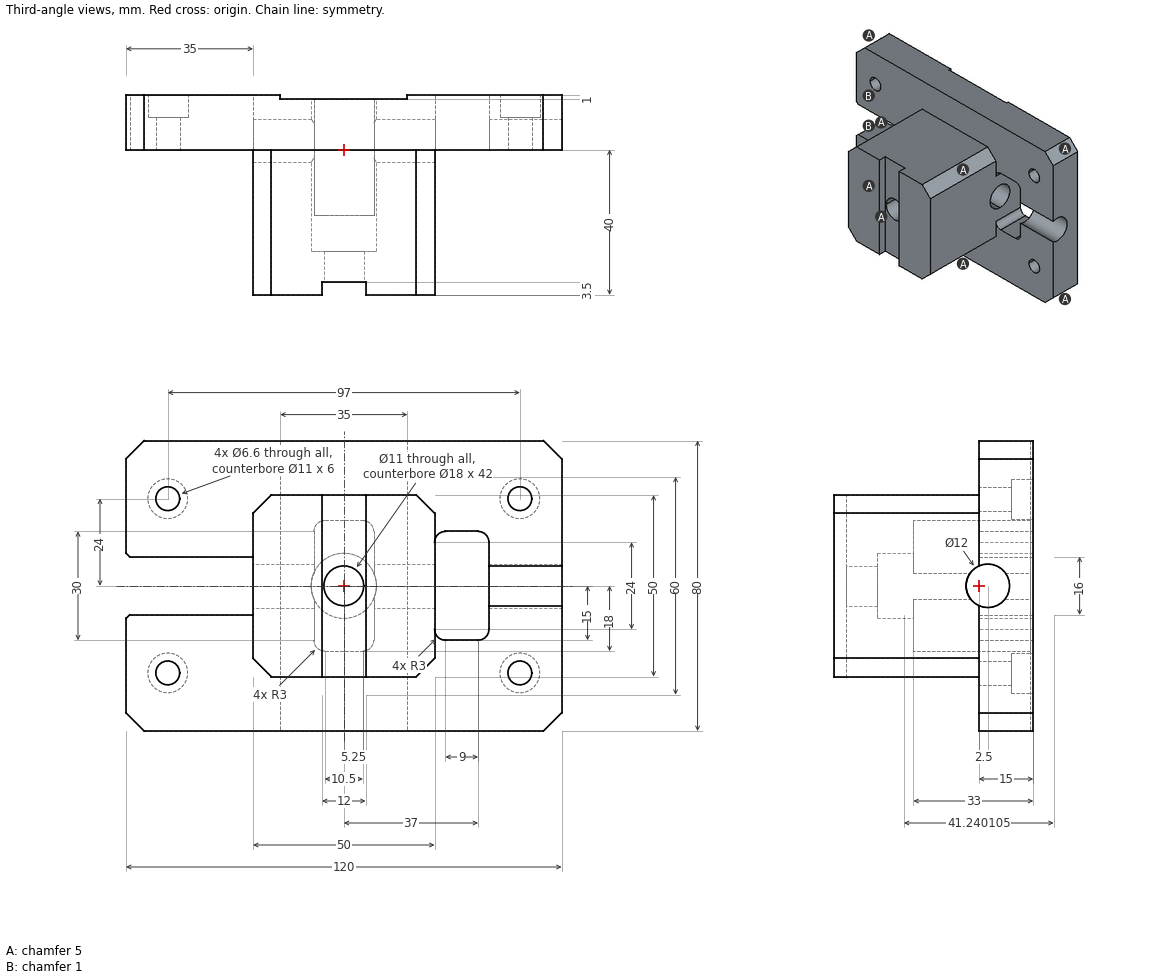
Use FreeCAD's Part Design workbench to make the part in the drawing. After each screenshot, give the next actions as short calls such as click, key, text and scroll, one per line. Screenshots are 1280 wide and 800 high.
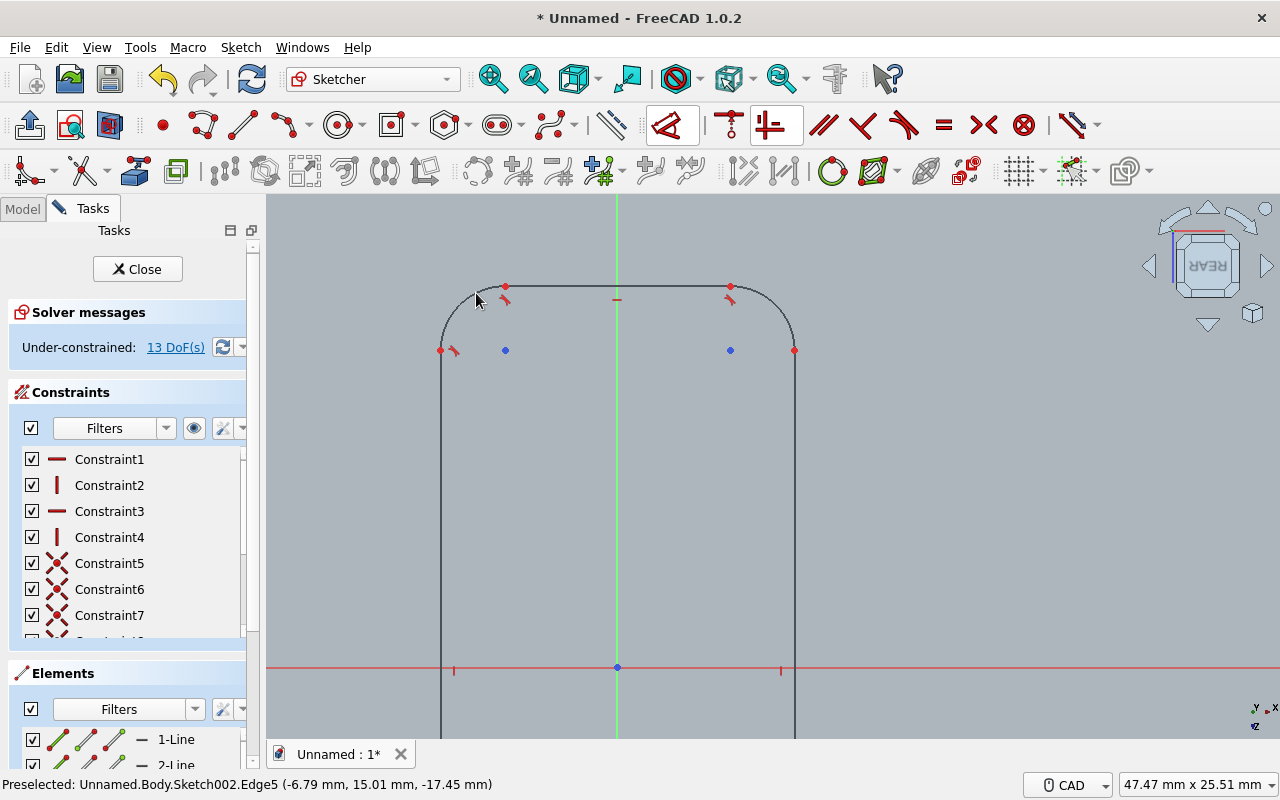
click(441, 542)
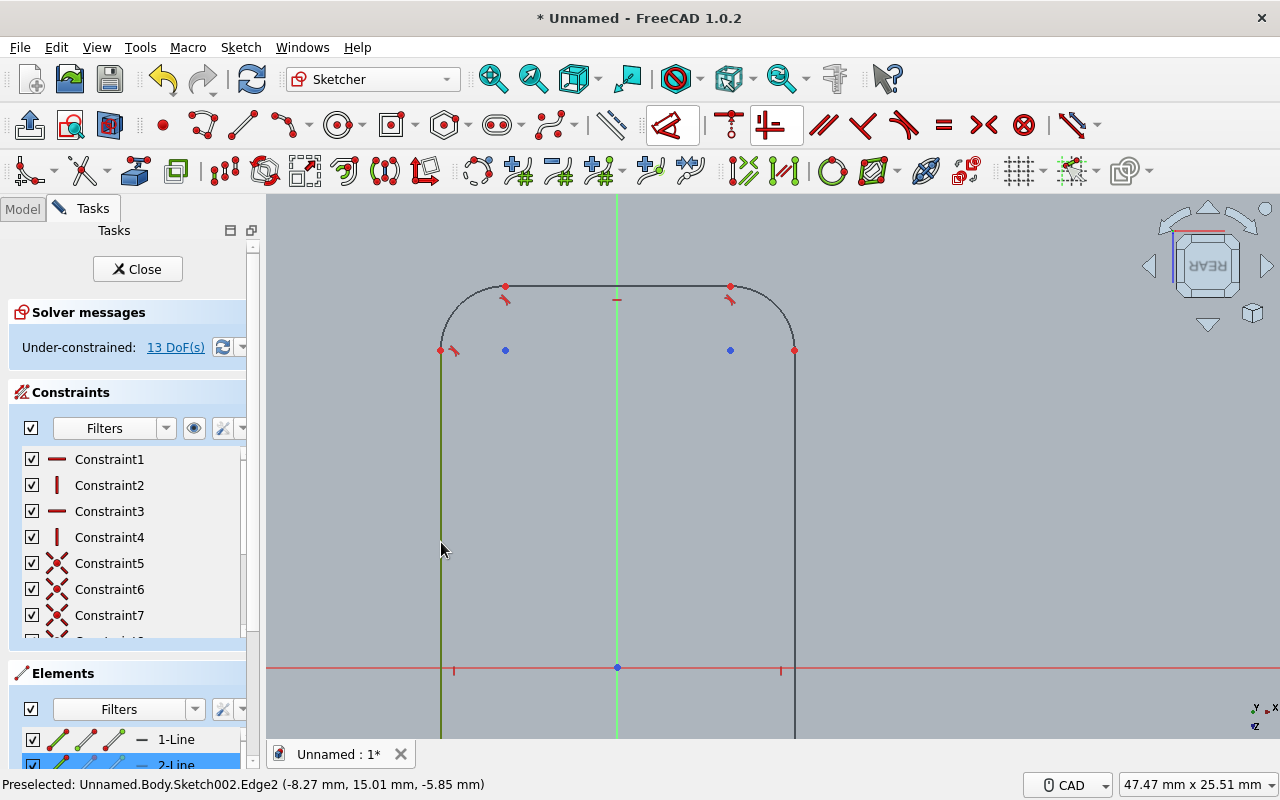
scroll(776, 302, down, 4)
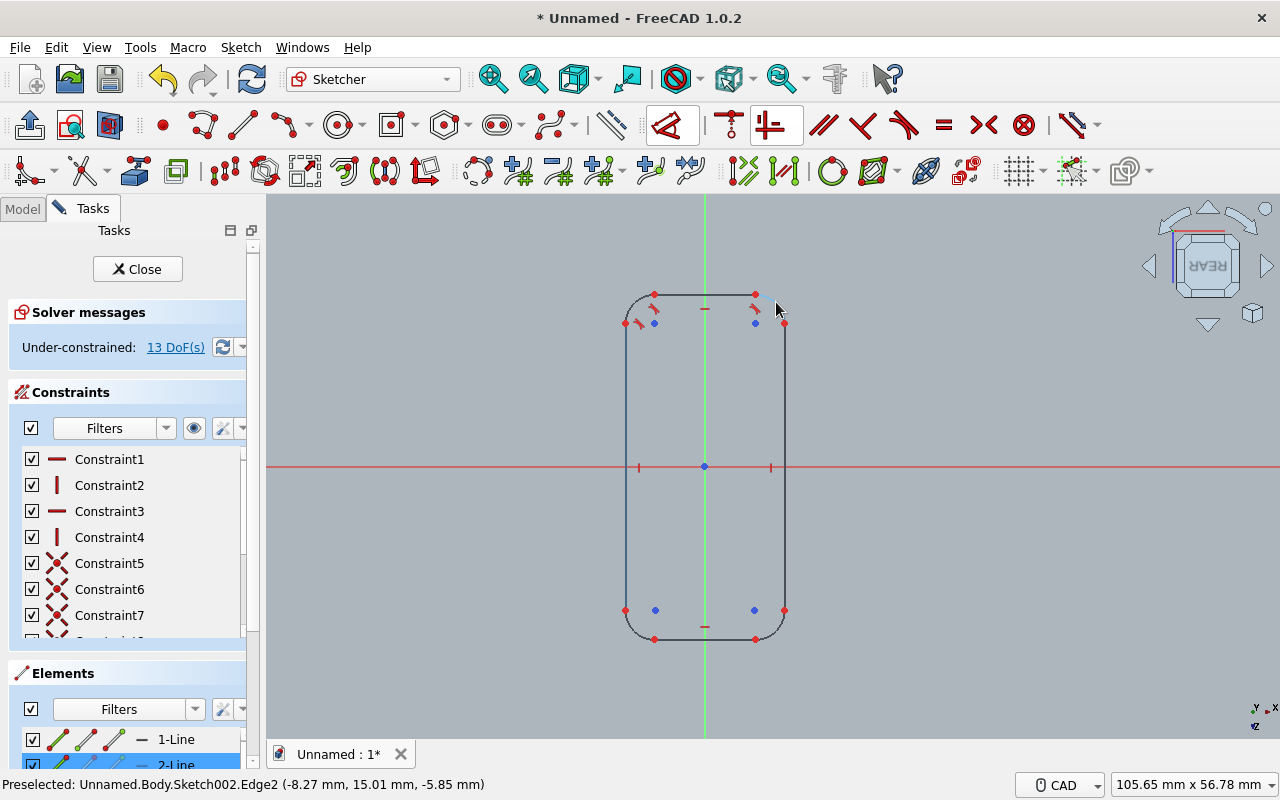
click(629, 624)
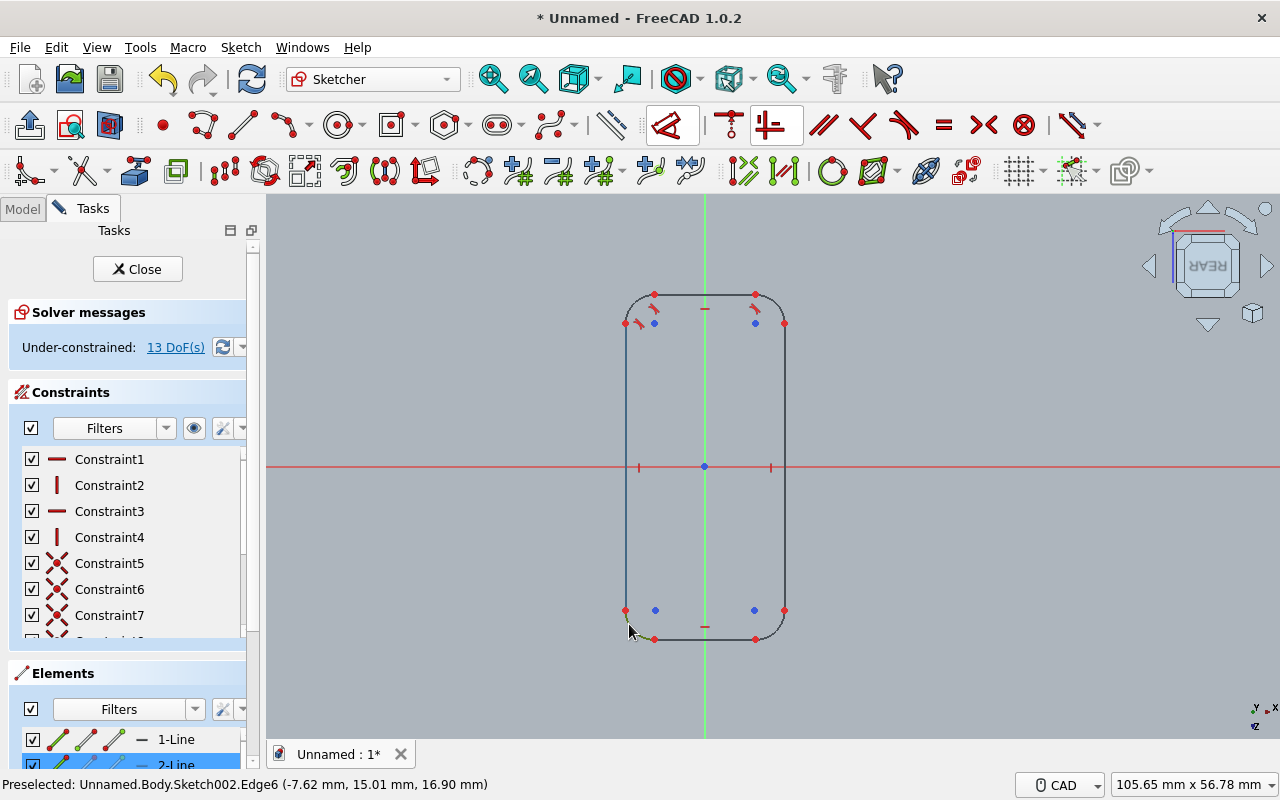
click(904, 126)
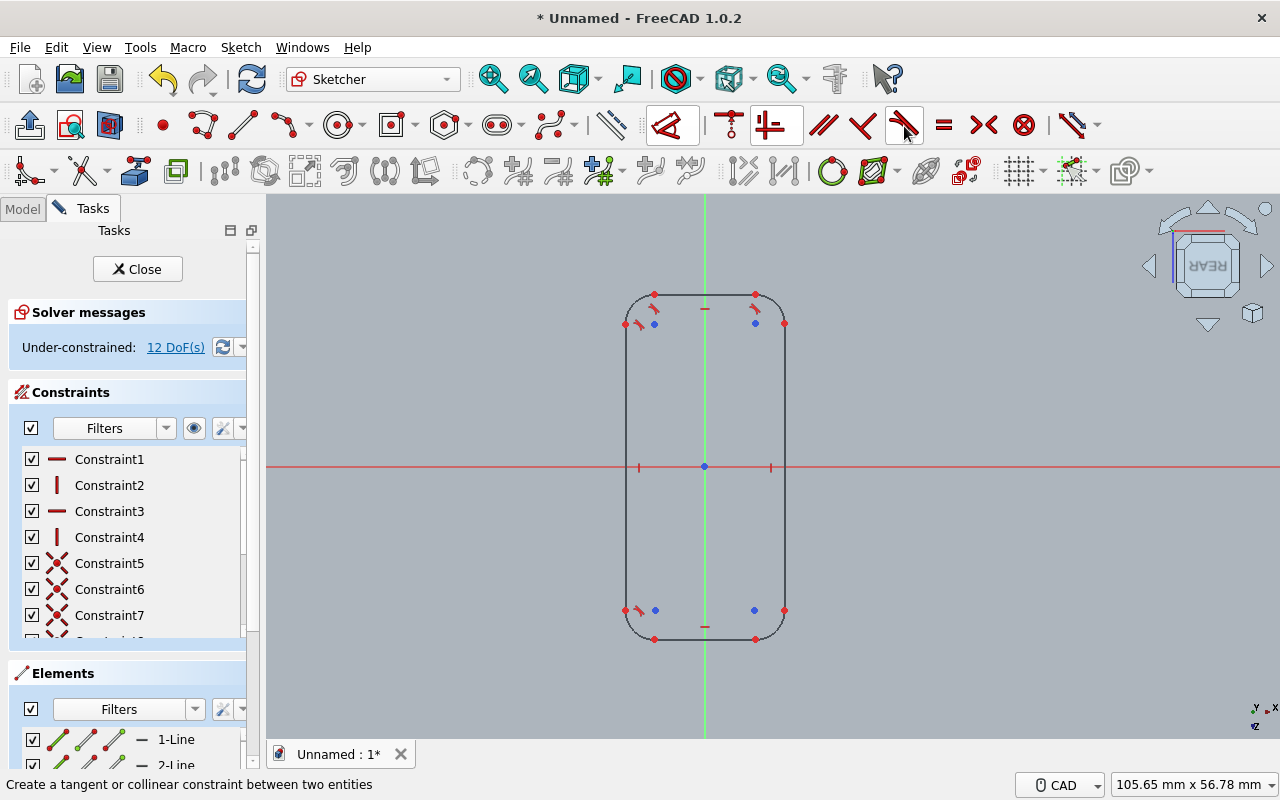
click(685, 640)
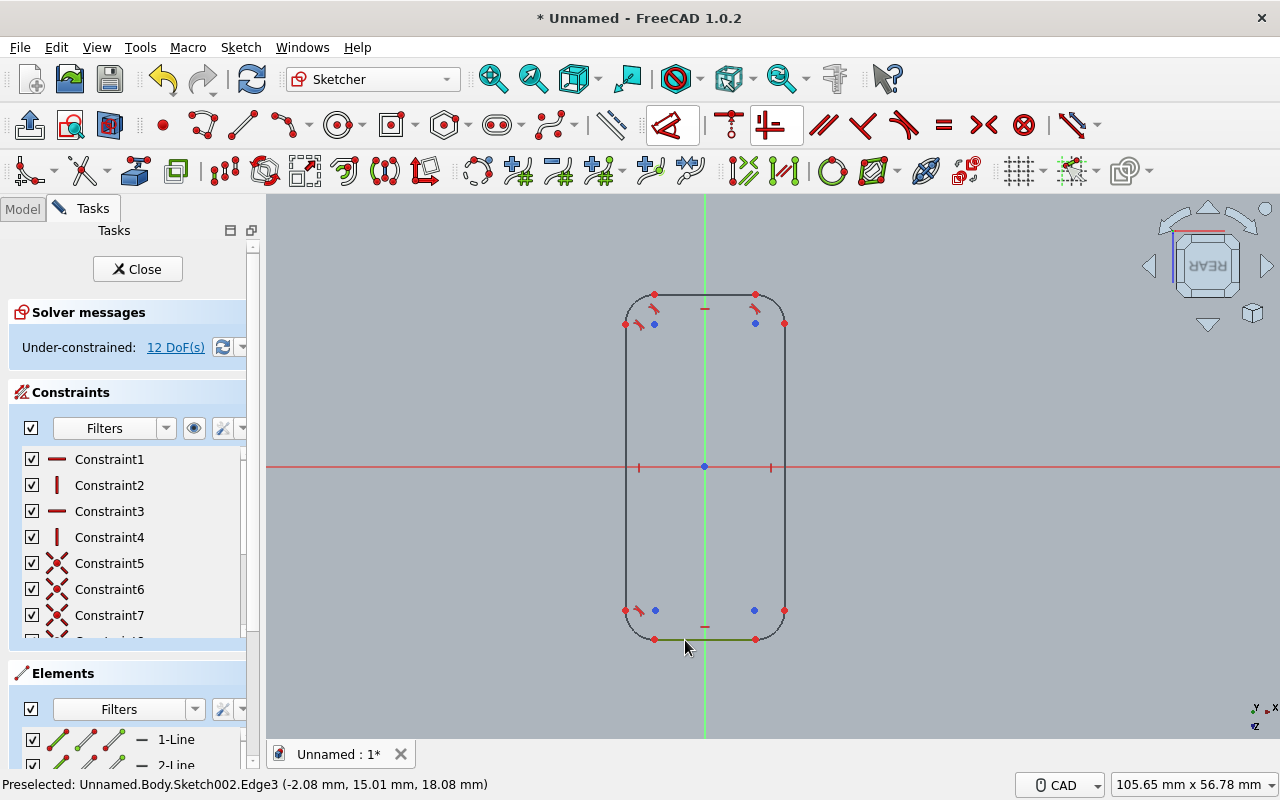
click(629, 624)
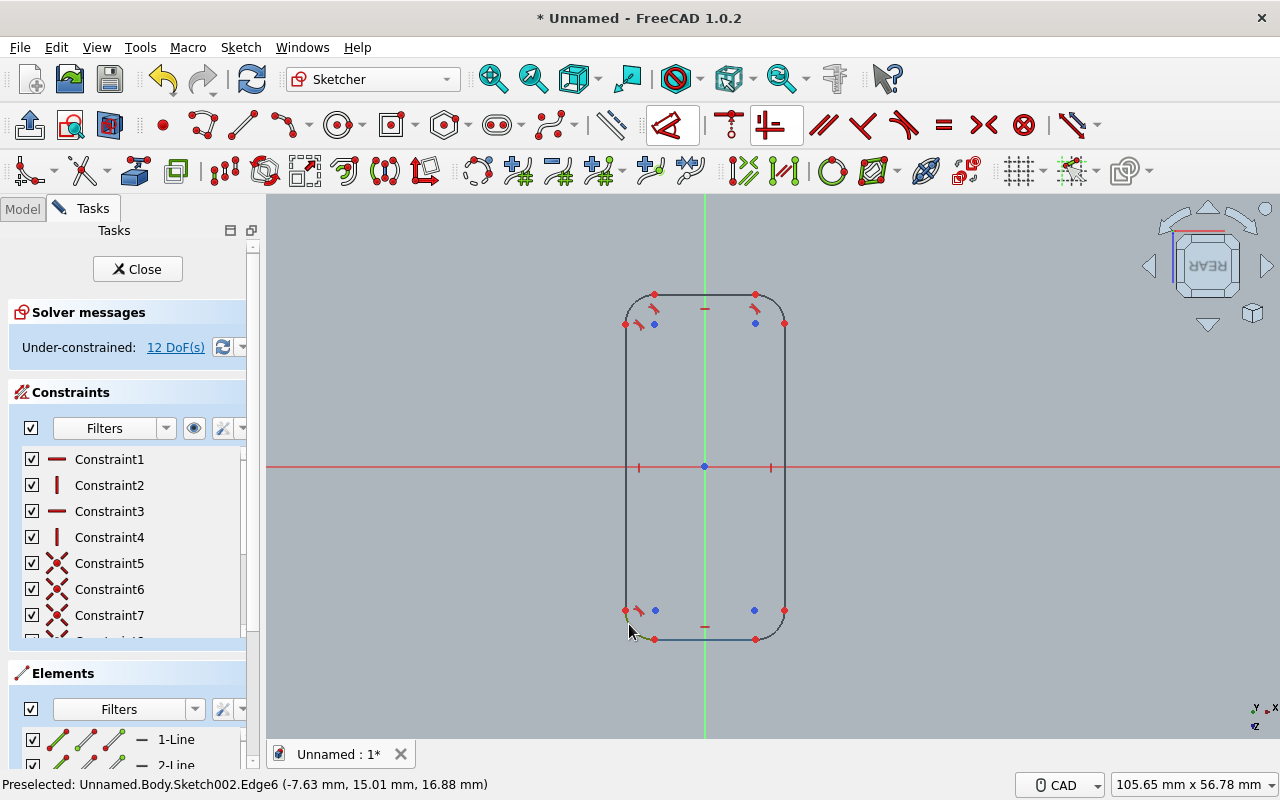
click(904, 126)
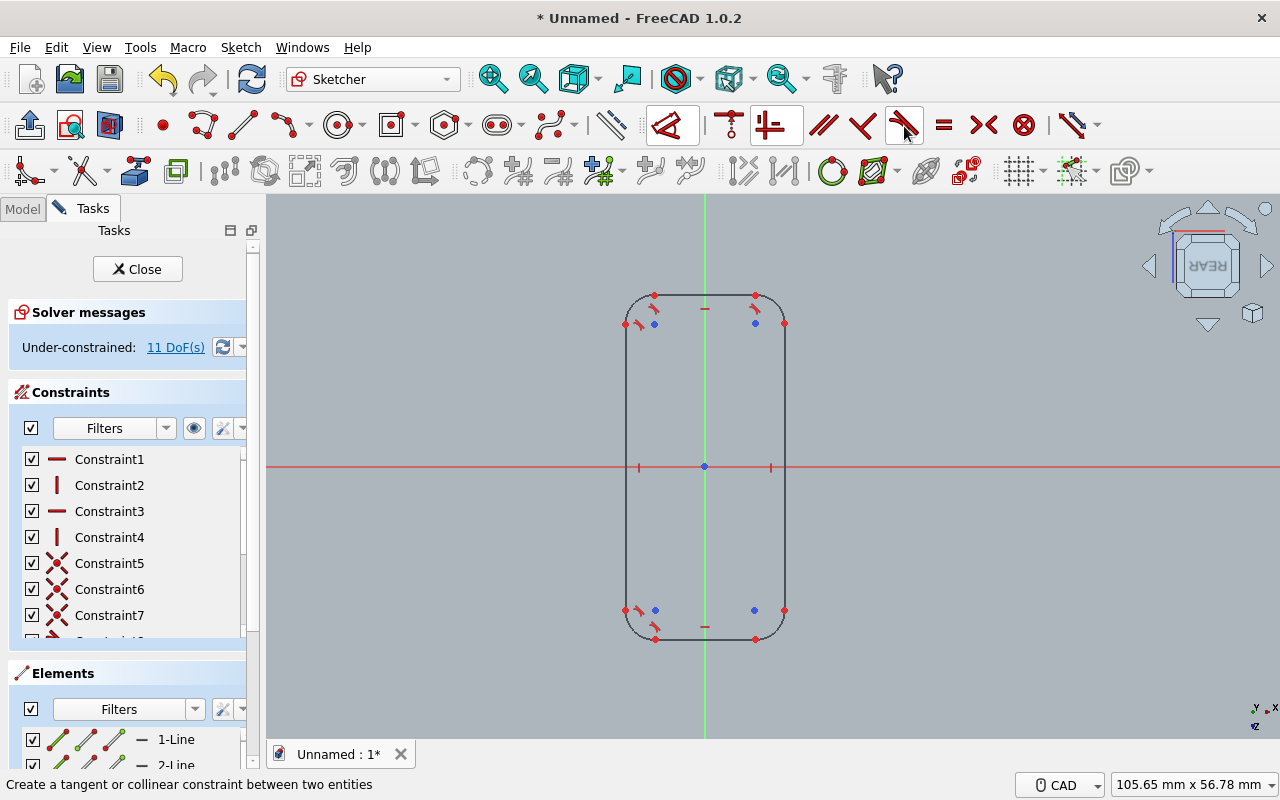
click(685, 640)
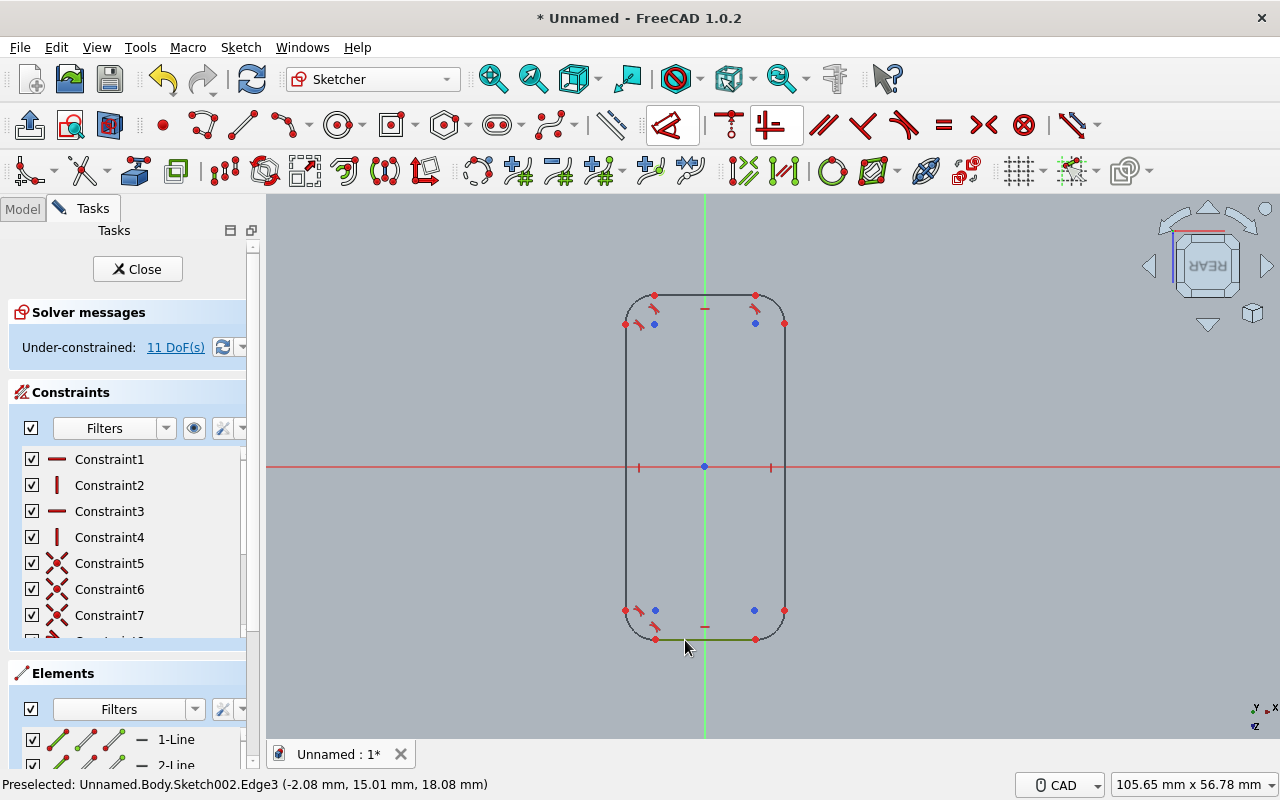
click(769, 637)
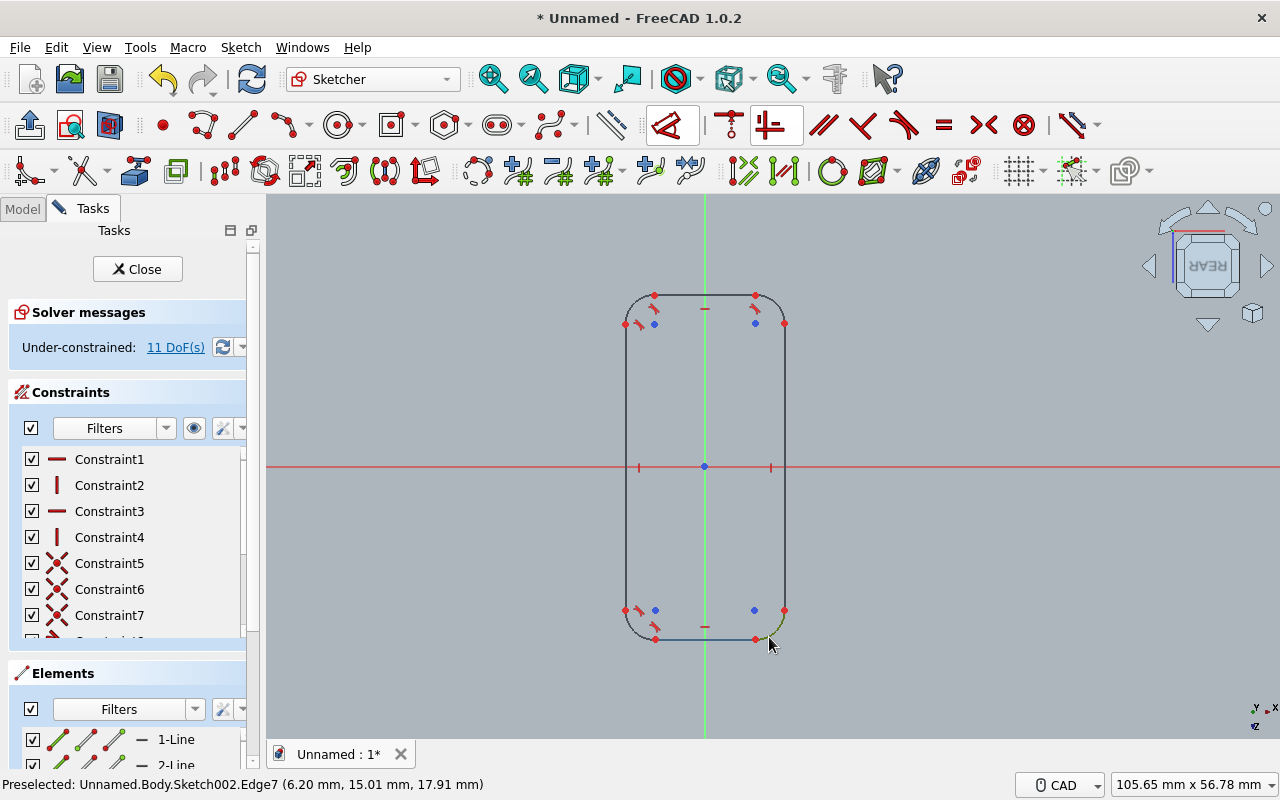
click(904, 126)